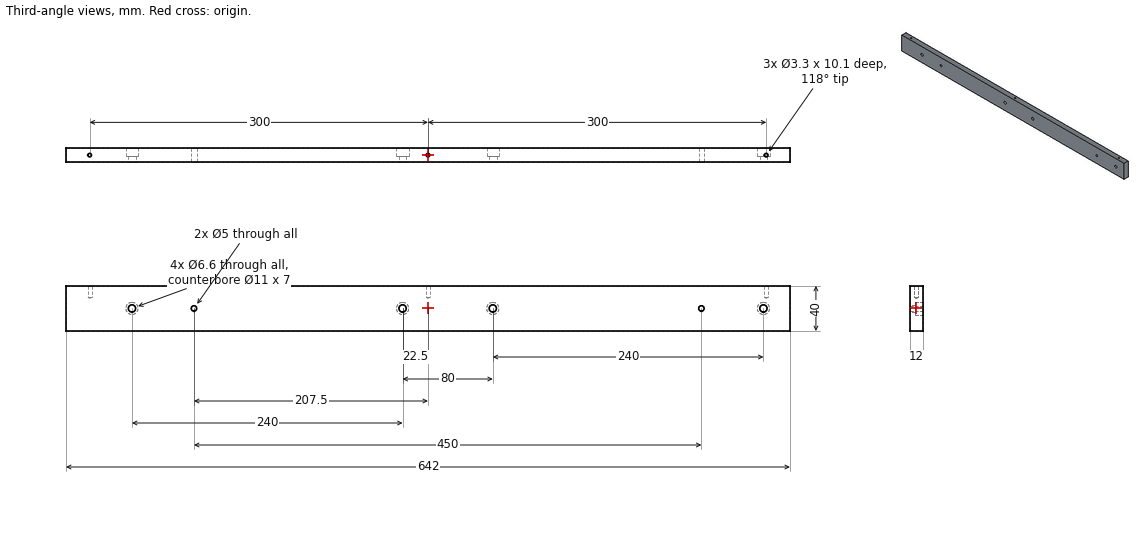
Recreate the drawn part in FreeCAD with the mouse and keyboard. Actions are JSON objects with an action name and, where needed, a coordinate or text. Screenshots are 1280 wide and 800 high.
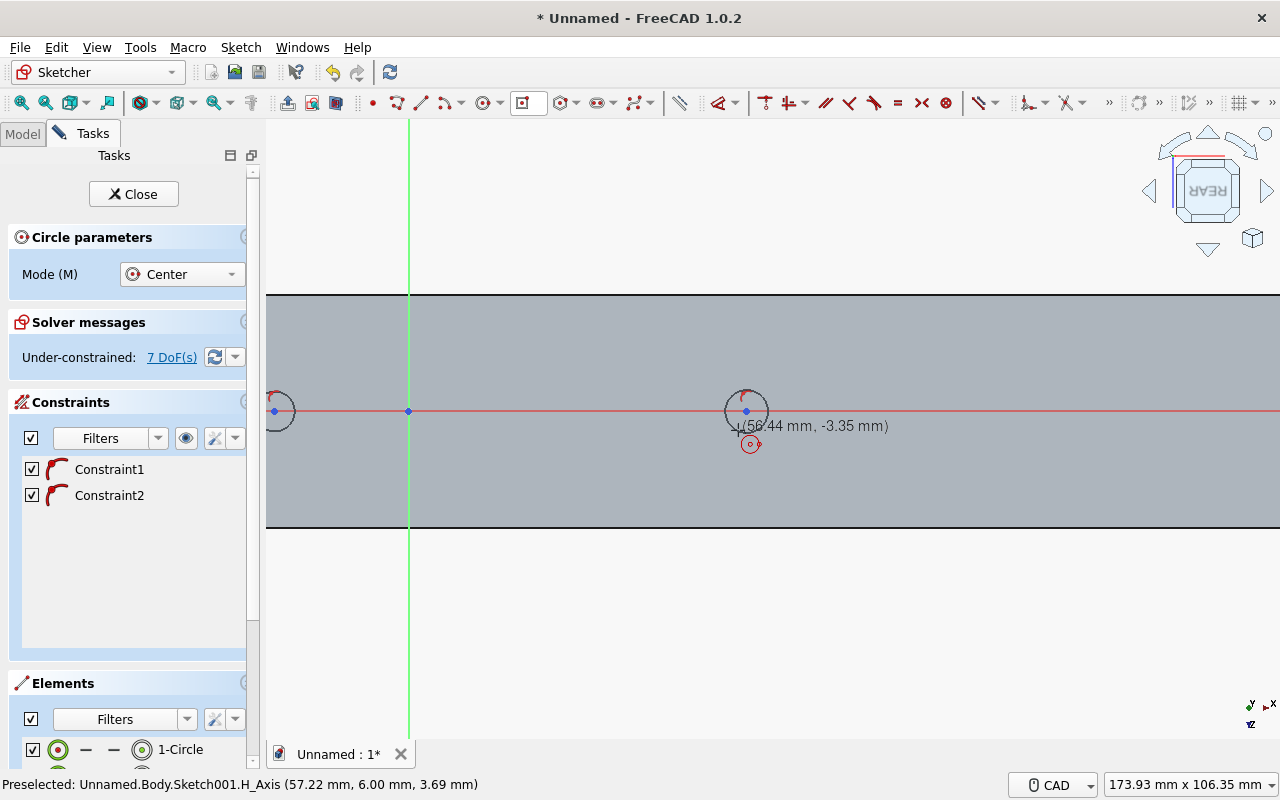
{"action": "scroll", "coordinate": [743, 432], "scroll_direction": "down", "scroll_amount": 9}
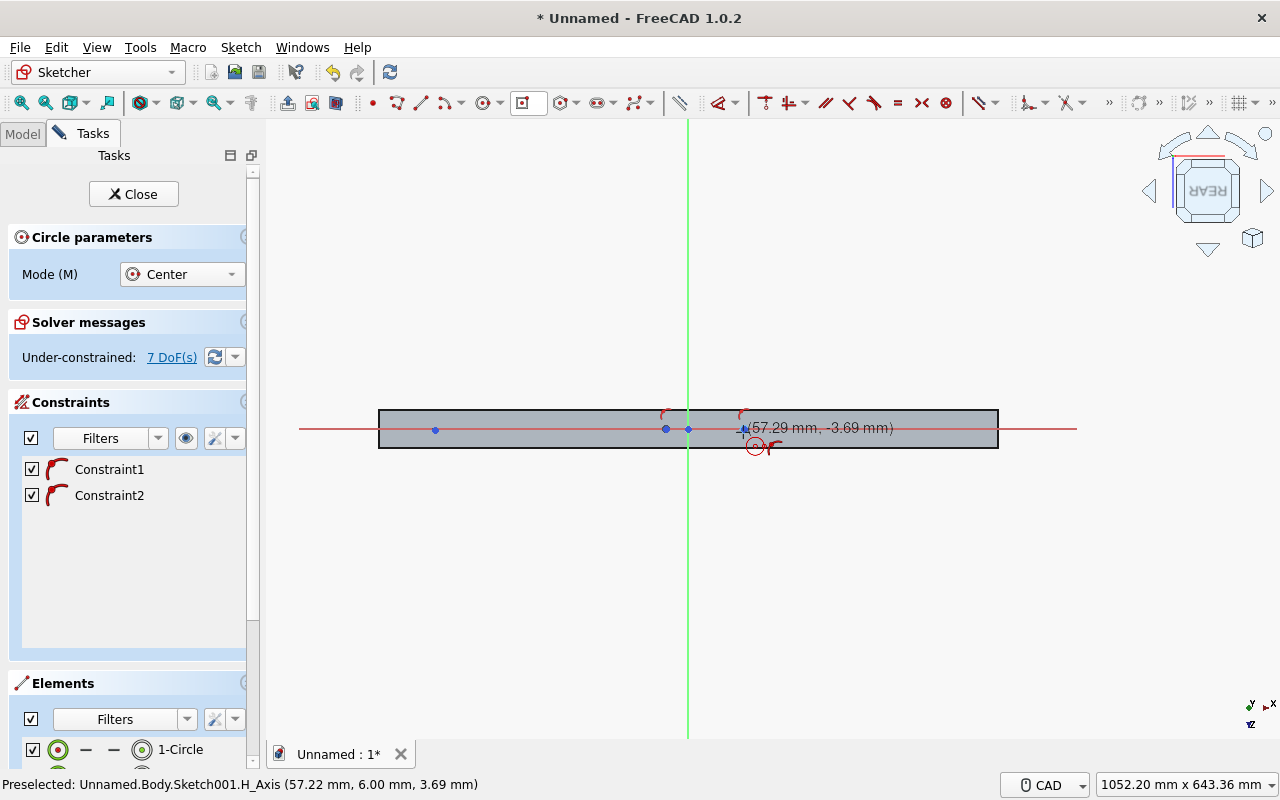
{"action": "scroll", "coordinate": [975, 429], "scroll_direction": "up", "scroll_amount": 10}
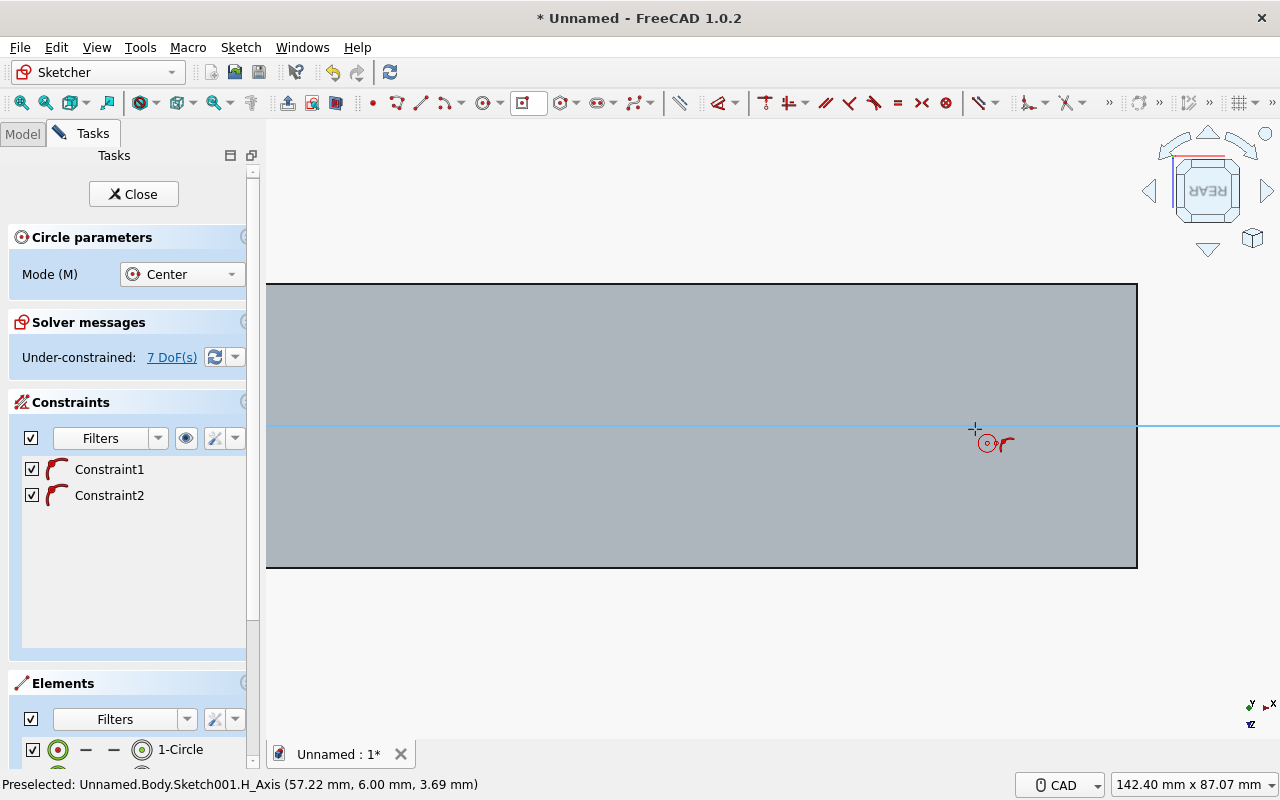
{"action": "scroll", "coordinate": [975, 429], "scroll_direction": "down", "scroll_amount": 10}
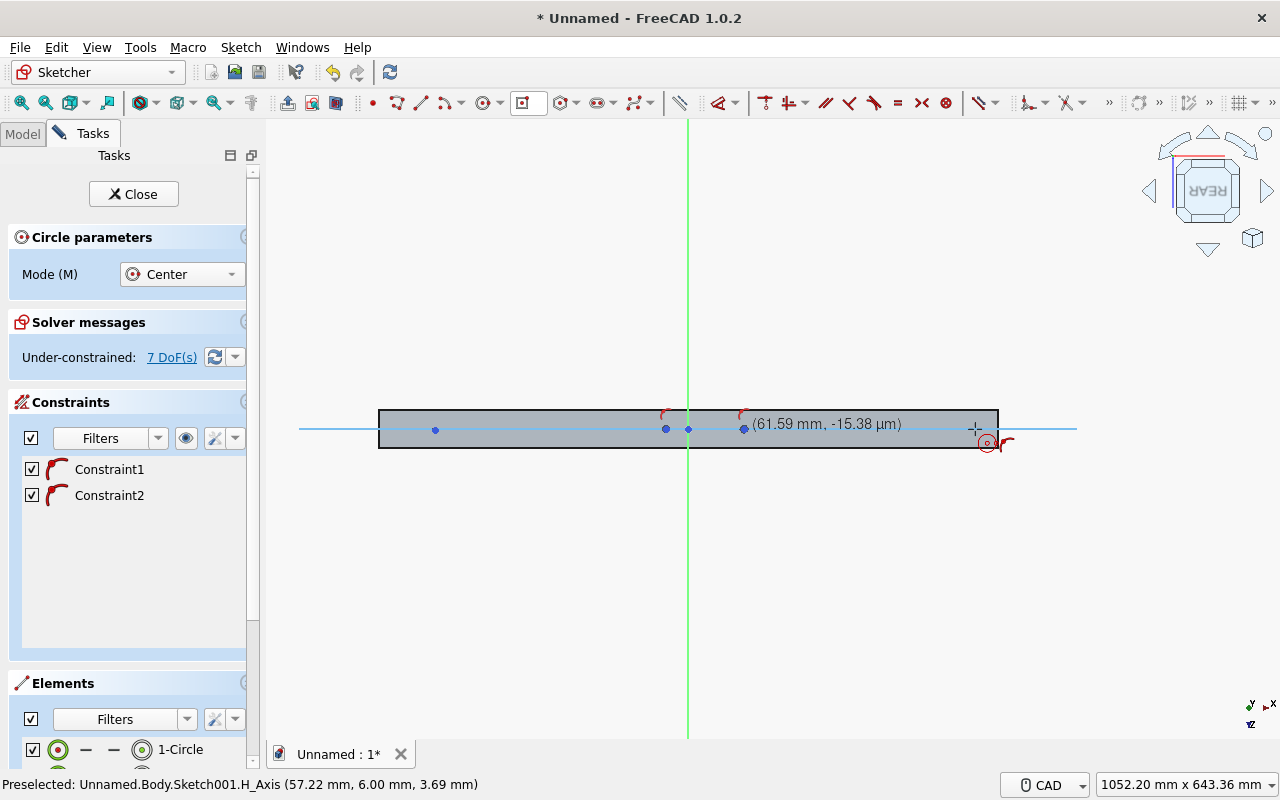
{"action": "left_click", "coordinate": [975, 429]}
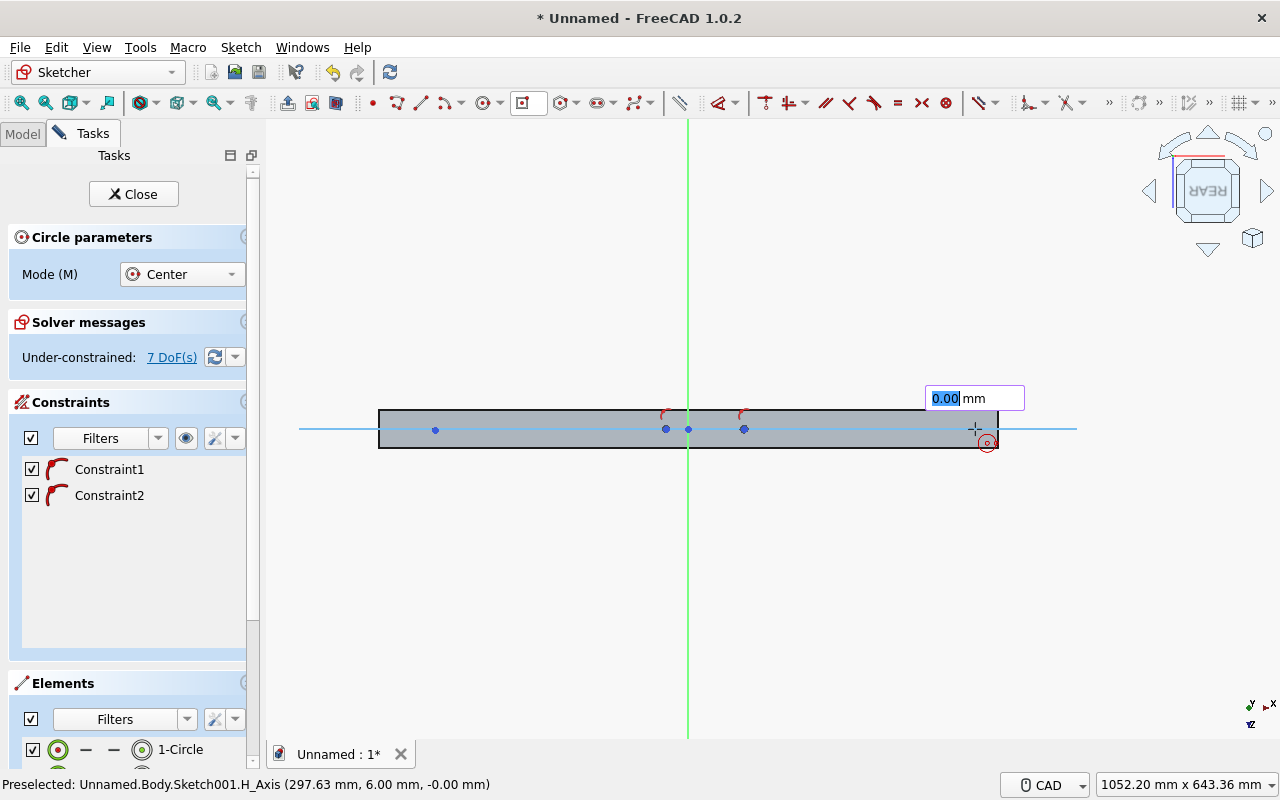
{"action": "scroll", "coordinate": [974, 432], "scroll_direction": "up", "scroll_amount": 9}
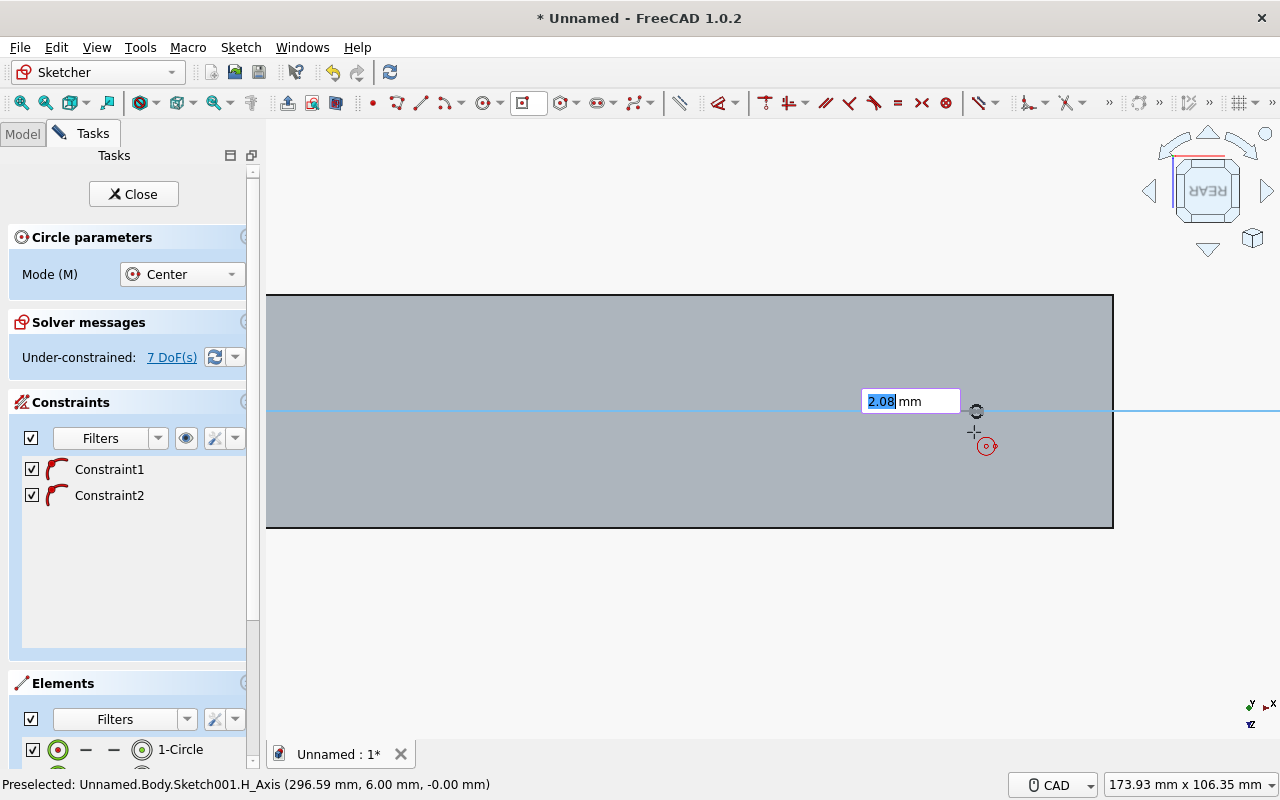
{"action": "left_click", "coordinate": [969, 430]}
{"action": "key", "text": "Escape"}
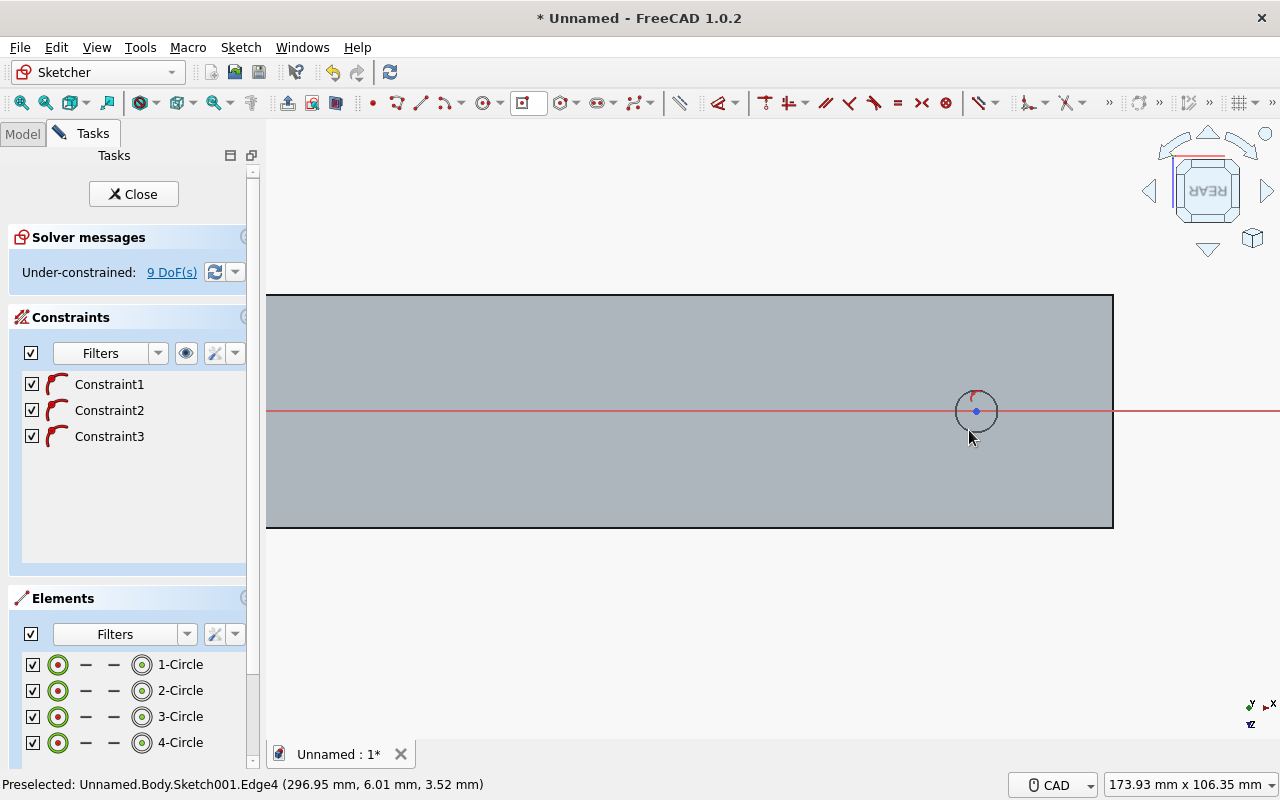
{"action": "scroll", "coordinate": [974, 432], "scroll_direction": "down", "scroll_amount": 9}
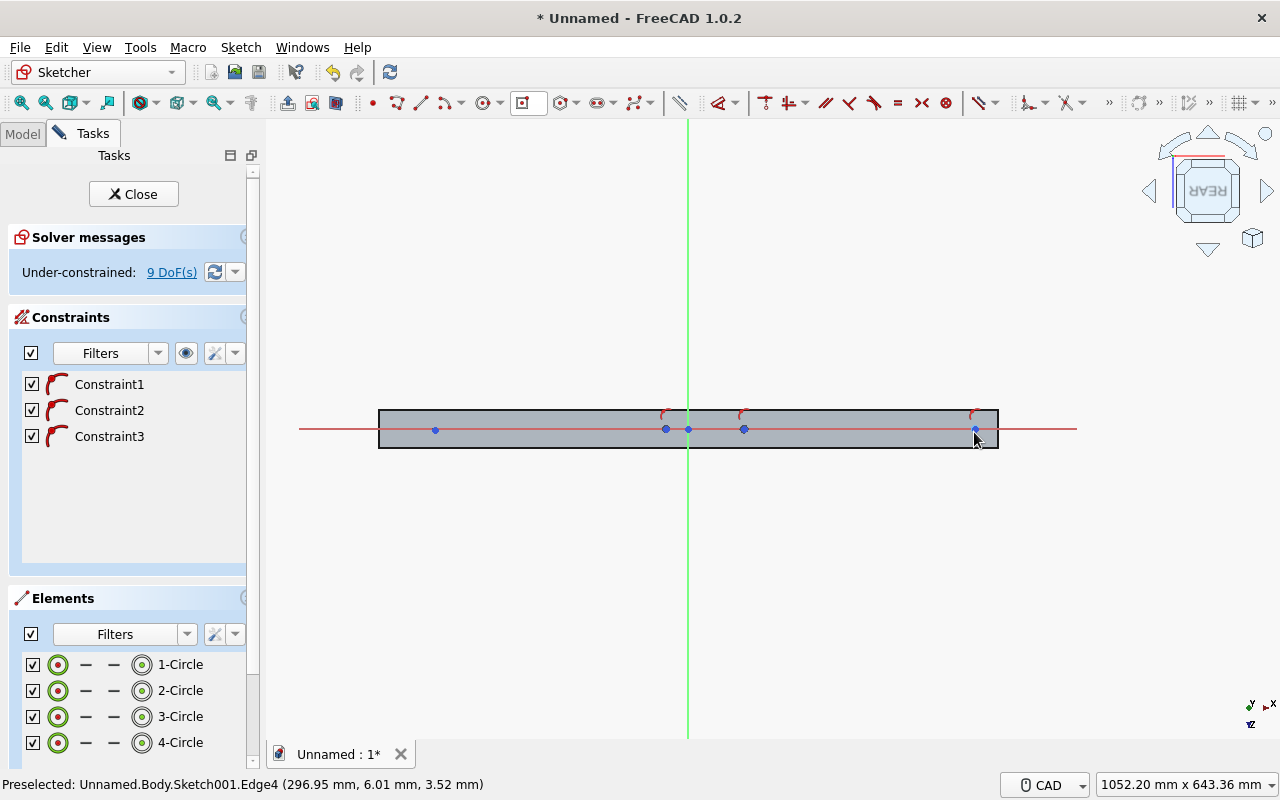
{"action": "scroll", "coordinate": [437, 429], "scroll_direction": "up", "scroll_amount": 10}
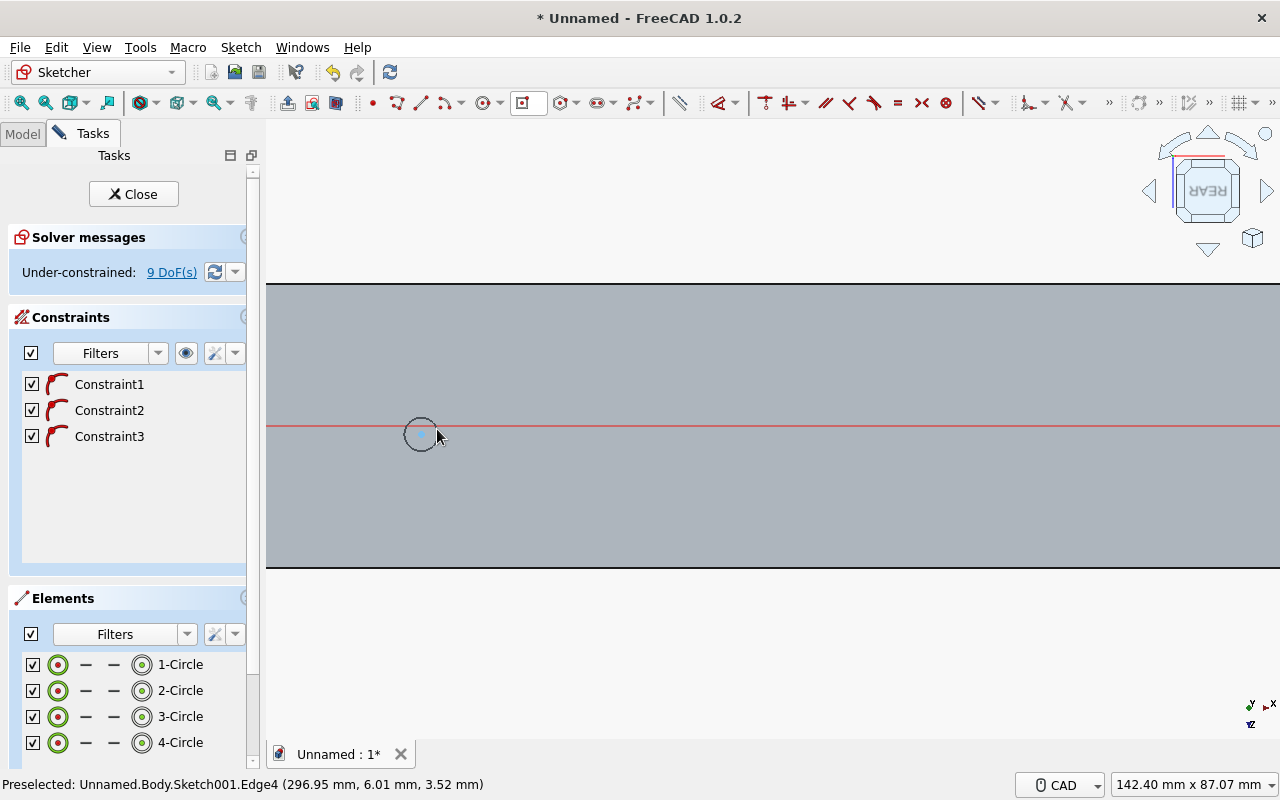
{"action": "left_click", "coordinate": [433, 423]}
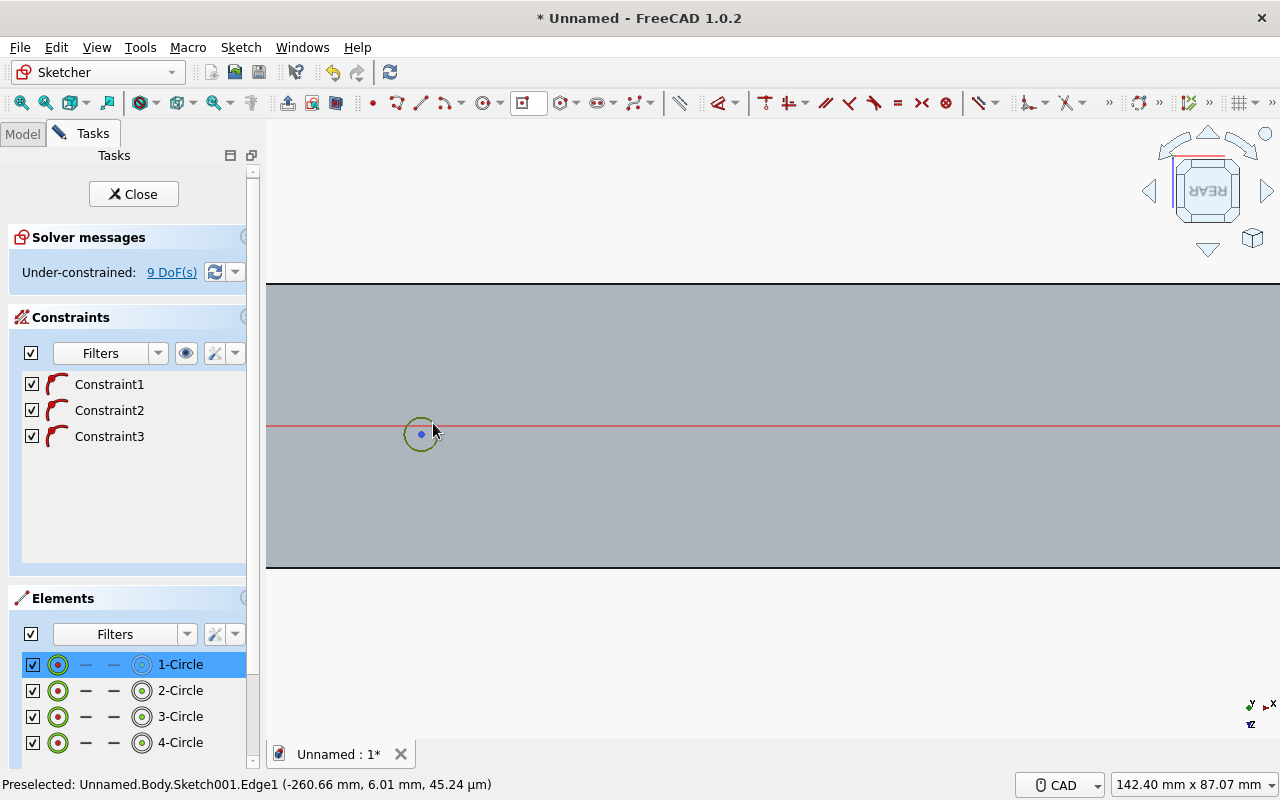
{"action": "scroll", "coordinate": [437, 429], "scroll_direction": "down", "scroll_amount": 10}